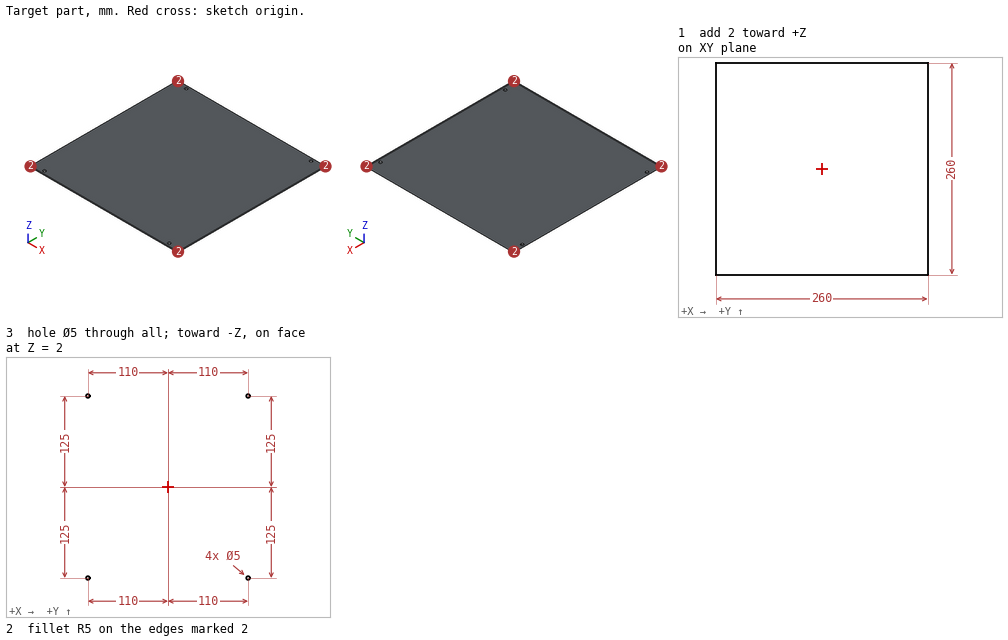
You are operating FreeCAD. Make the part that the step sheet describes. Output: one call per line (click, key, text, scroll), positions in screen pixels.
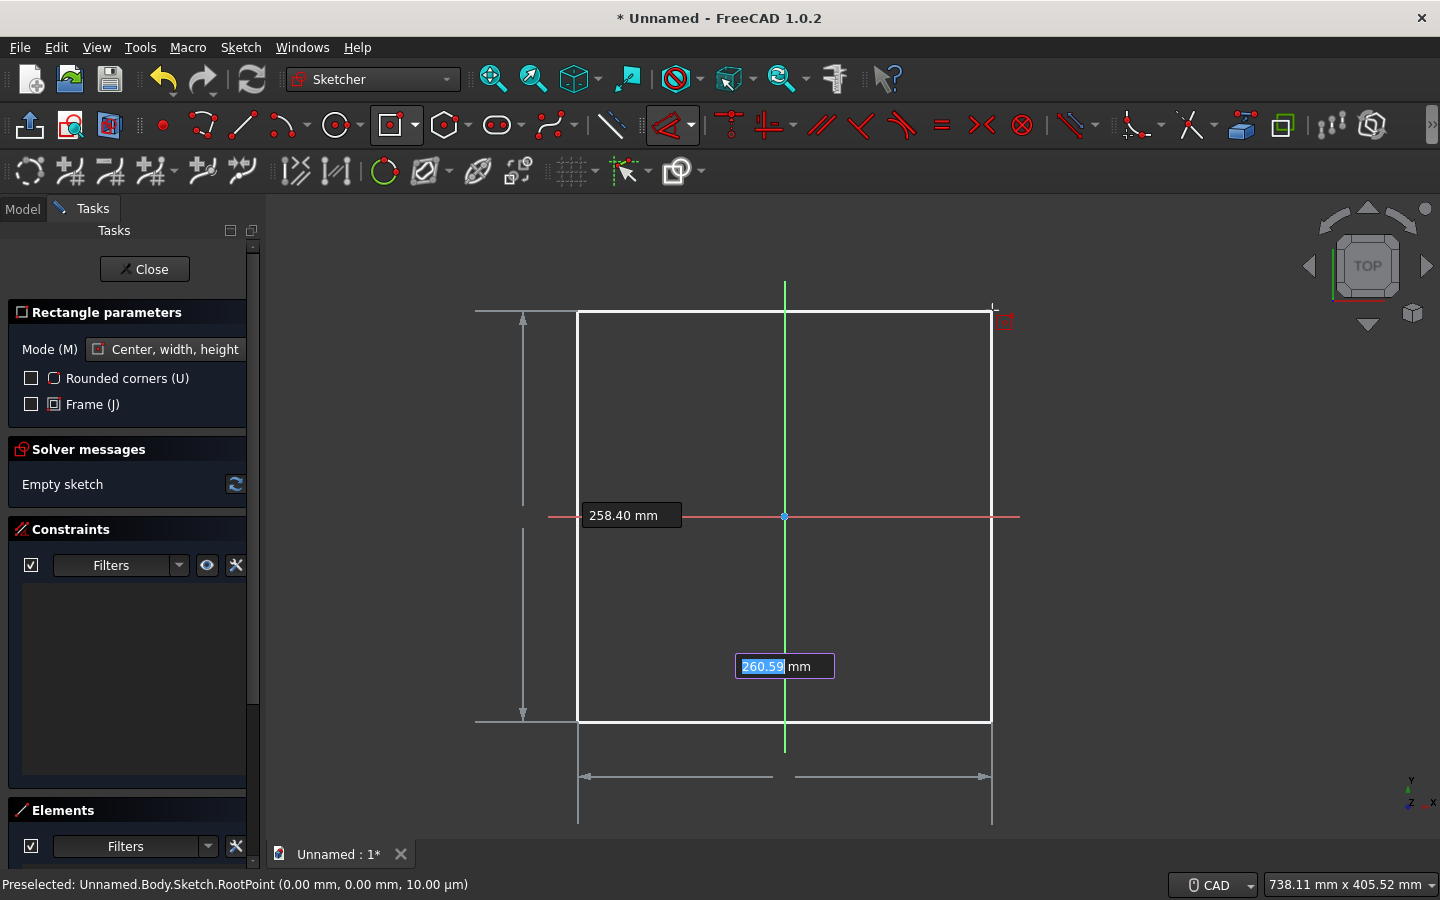
text(260)
key(Tab)
text(260)
key(Return)
key(Escape)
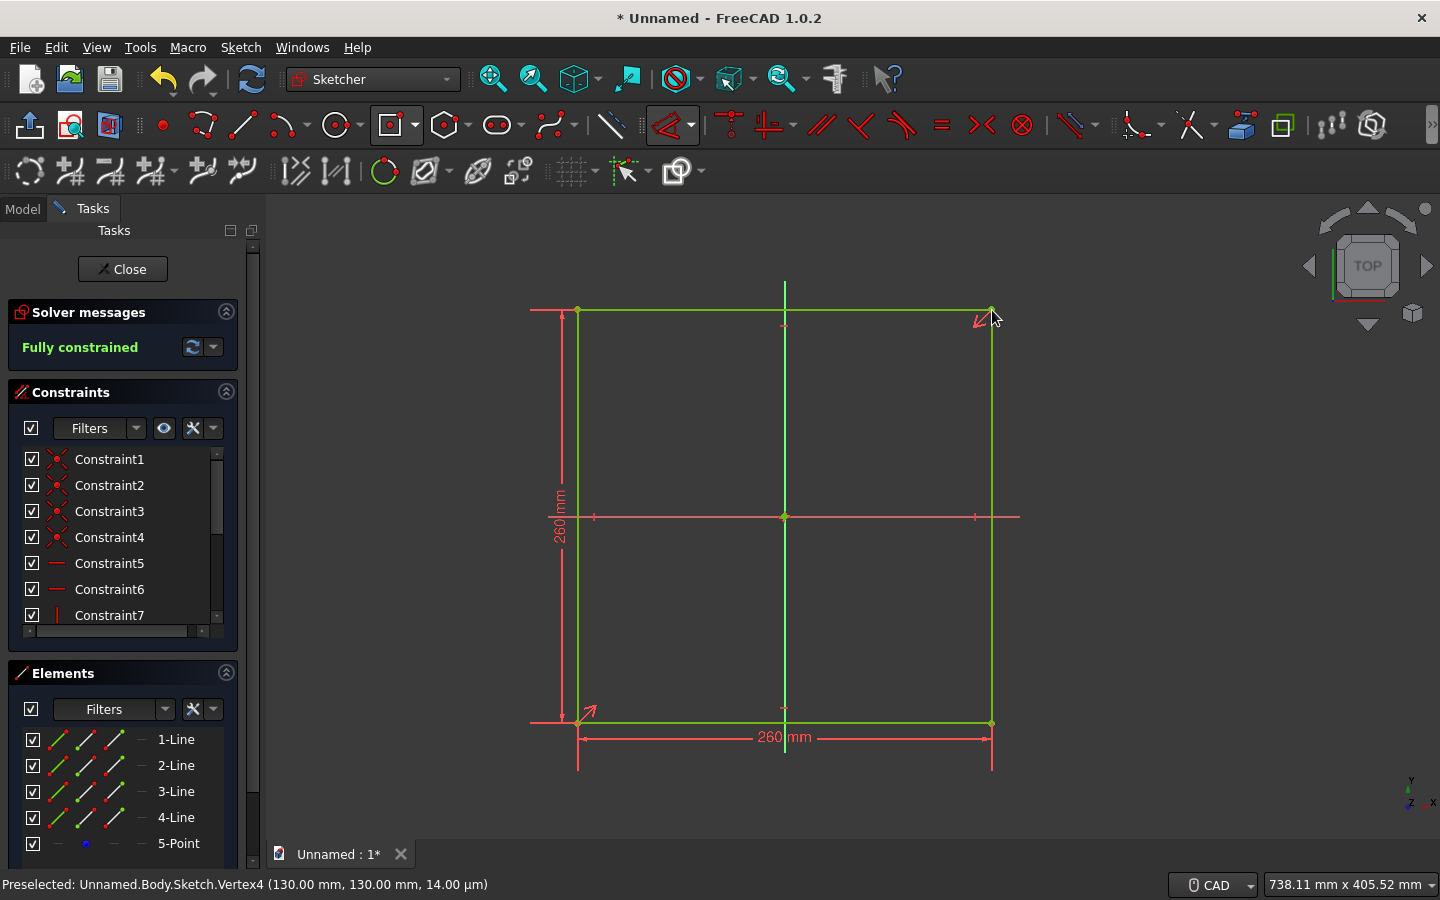
click(123, 269)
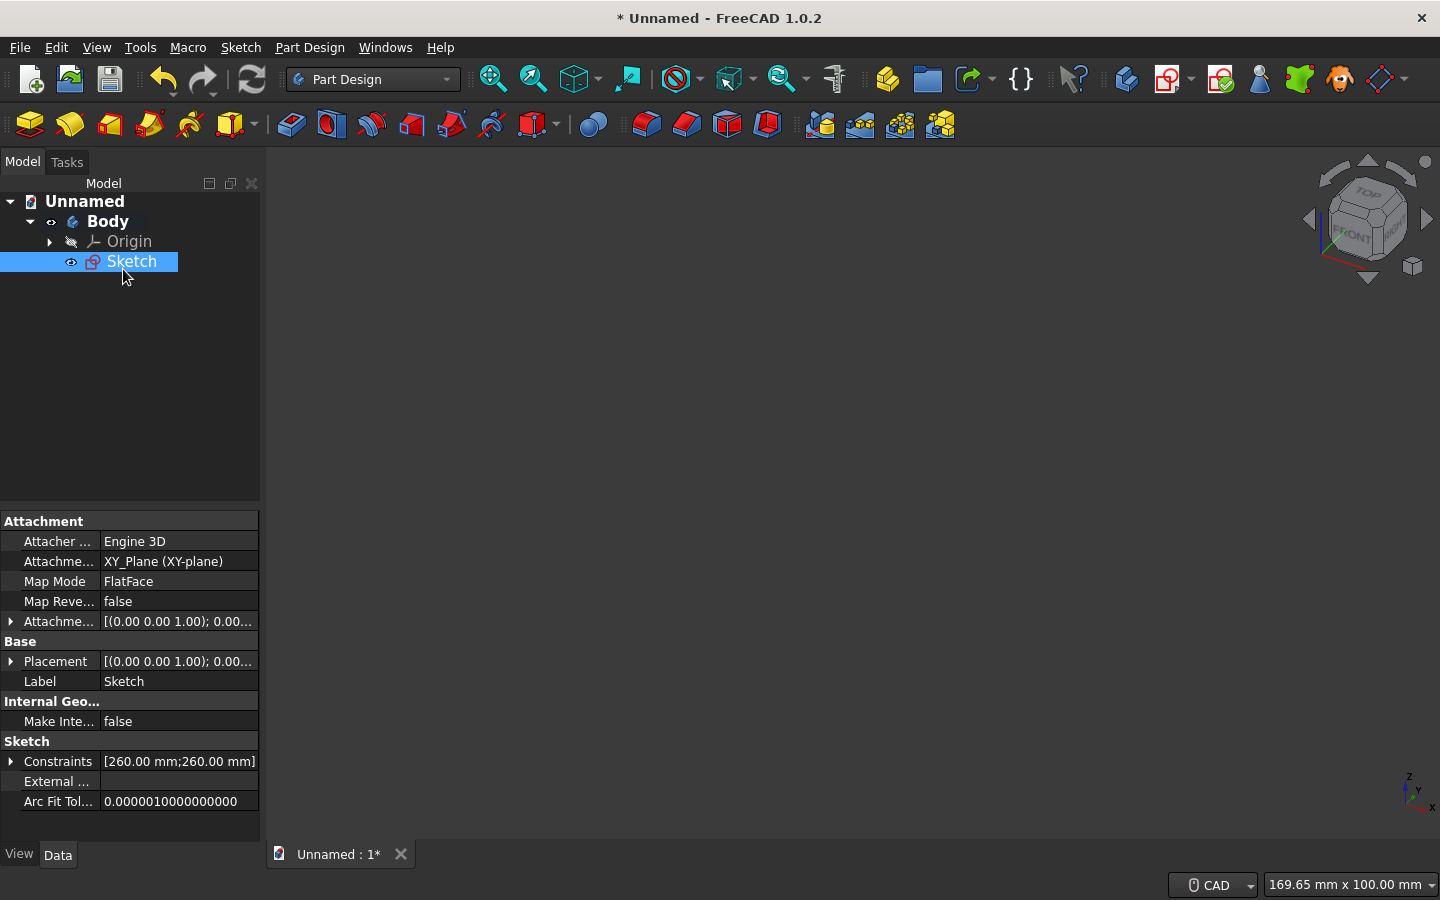
click(30, 124)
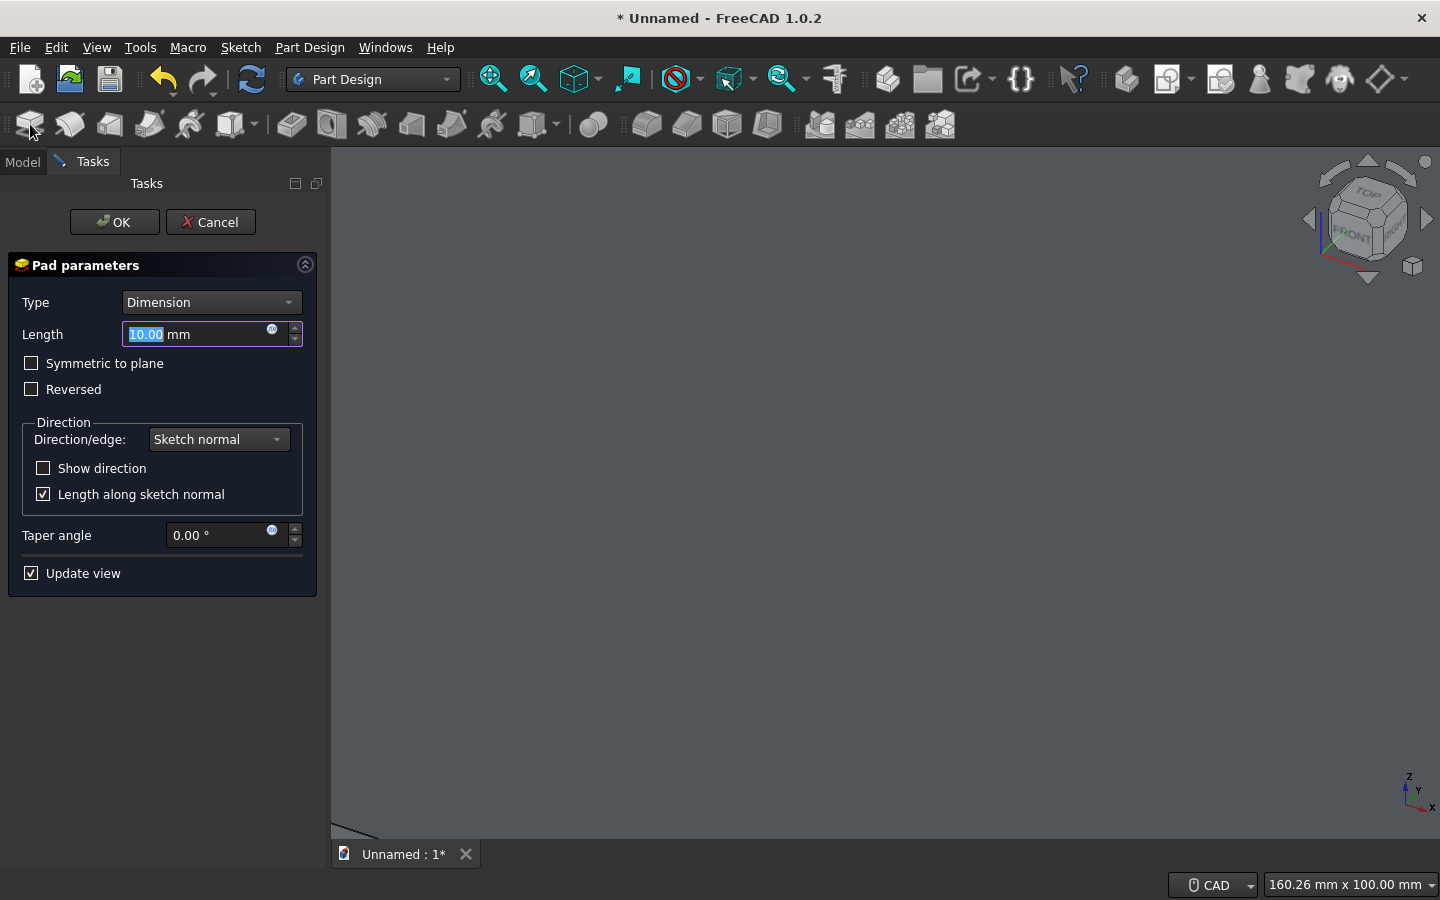
text(2)
key(Tab)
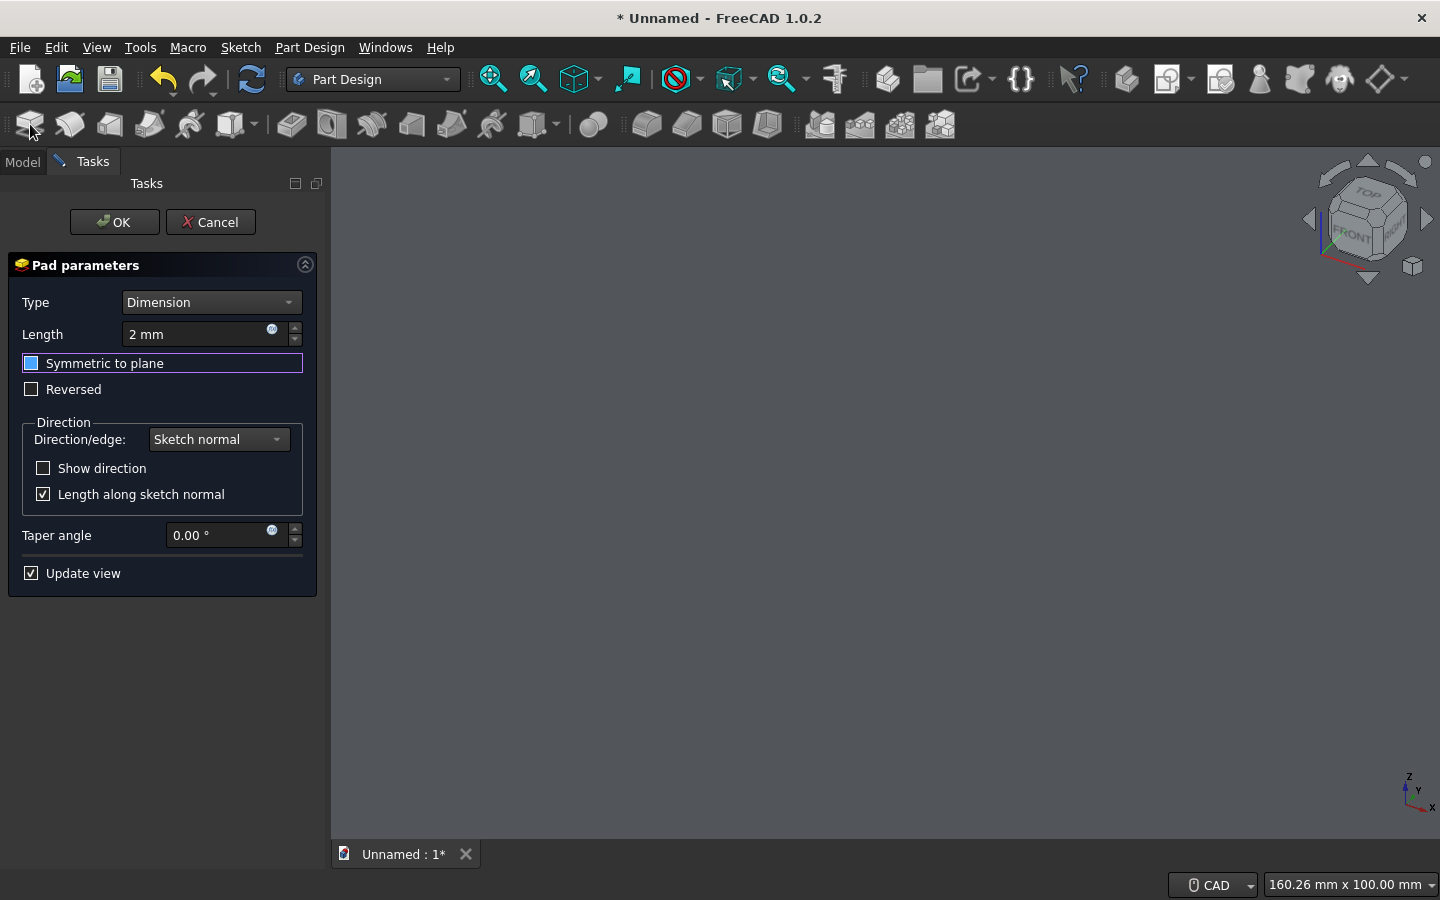
click(115, 222)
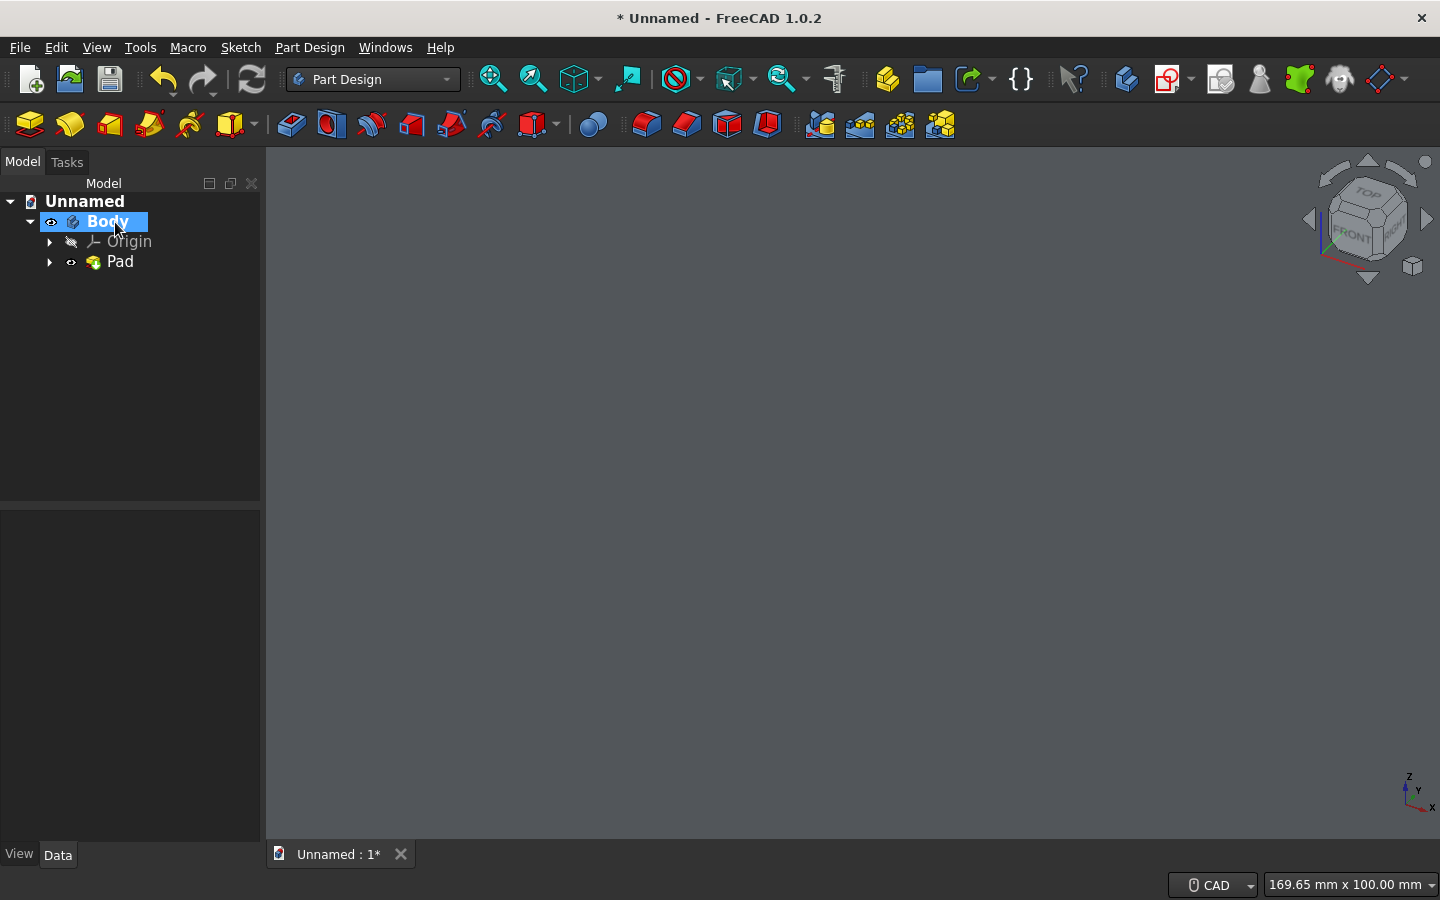
click(494, 80)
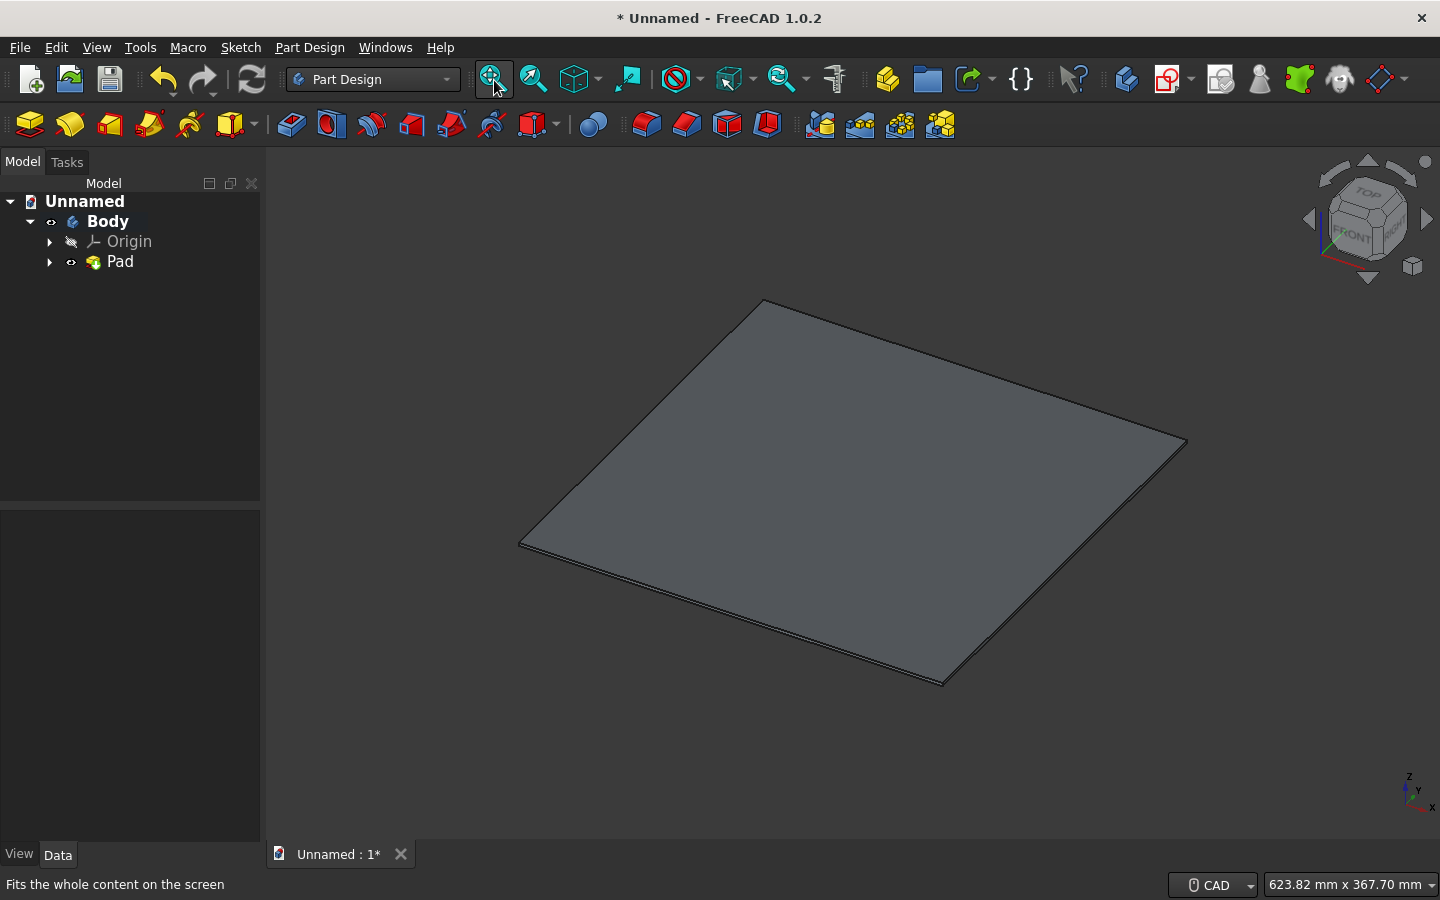
scroll(943, 684, up, 12)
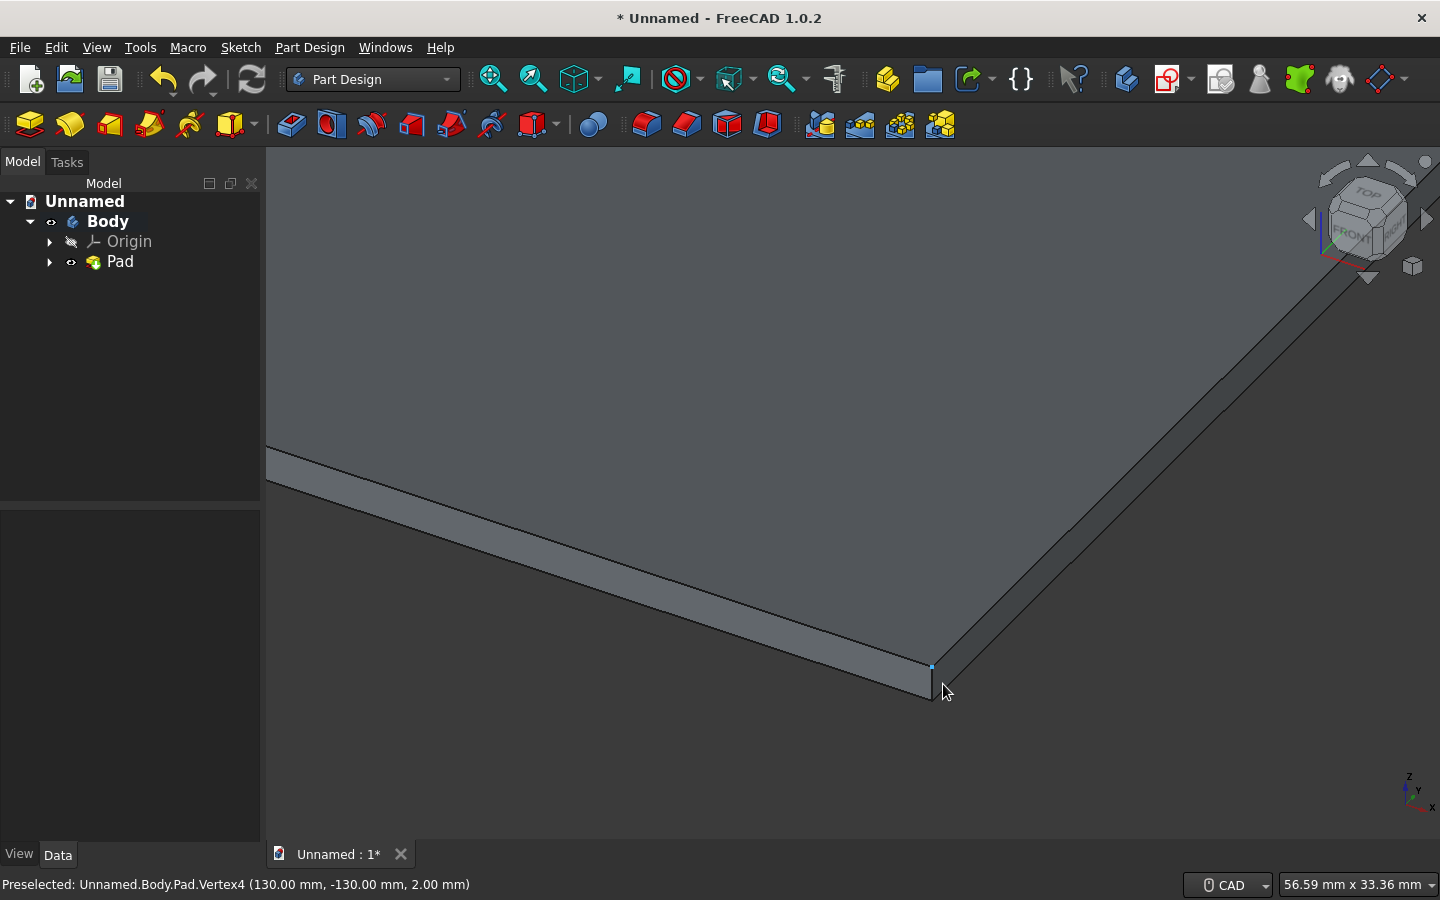
click(932, 683)